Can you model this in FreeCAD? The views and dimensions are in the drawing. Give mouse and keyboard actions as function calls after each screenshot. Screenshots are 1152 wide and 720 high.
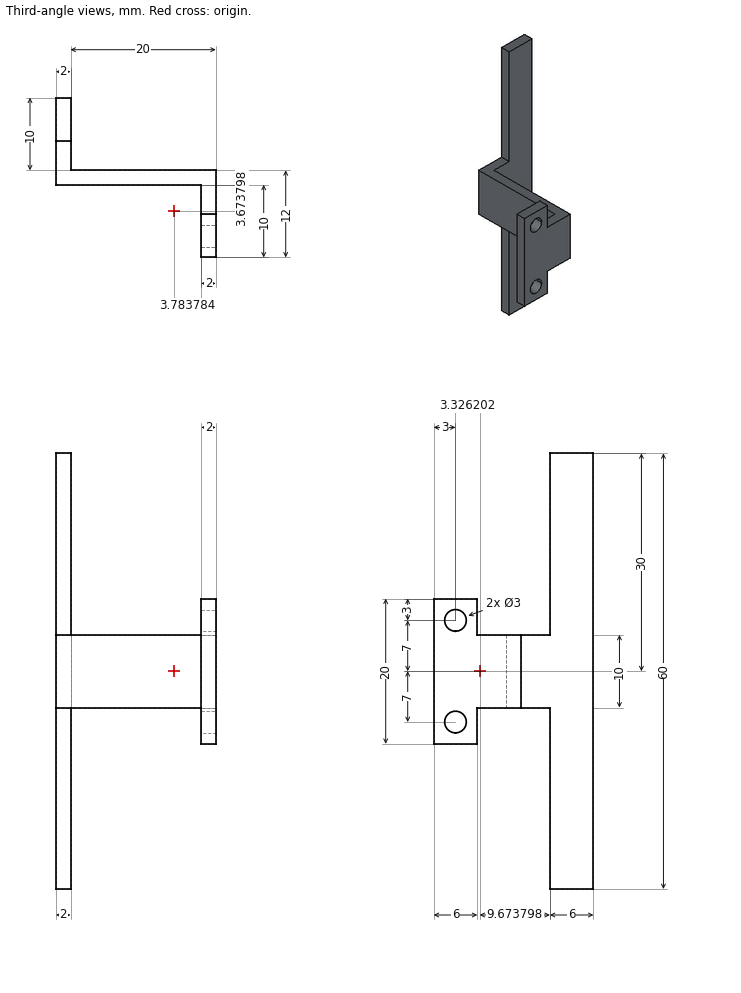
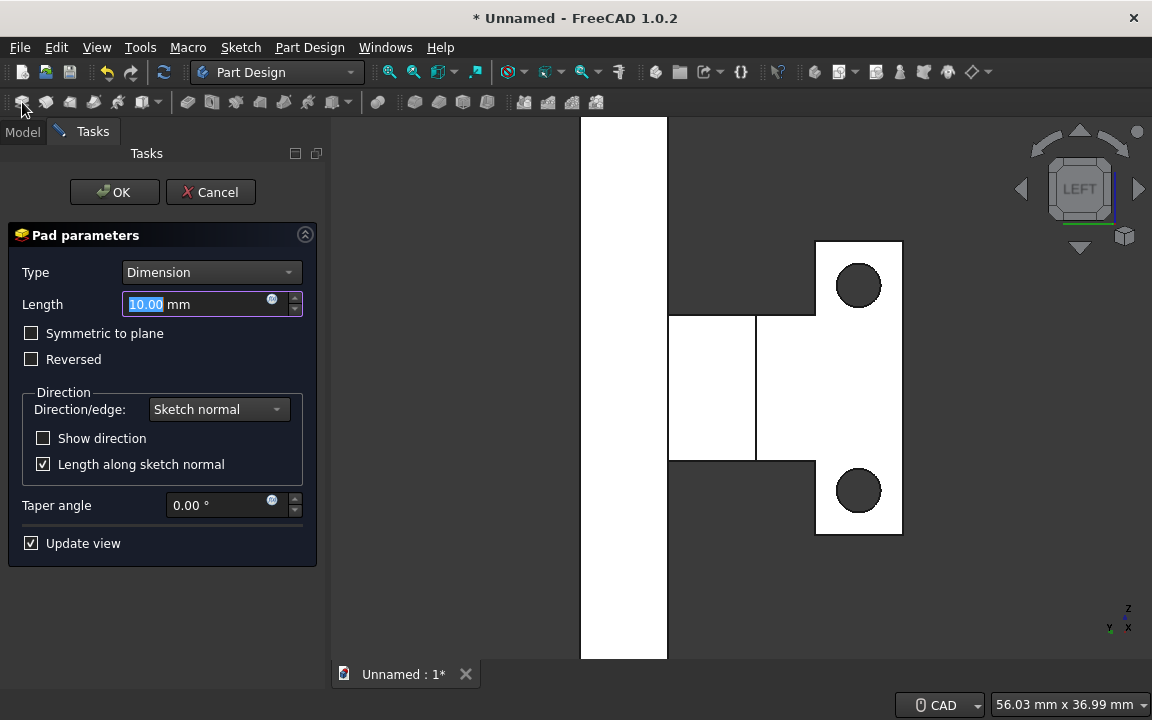
text(2)
key(Tab)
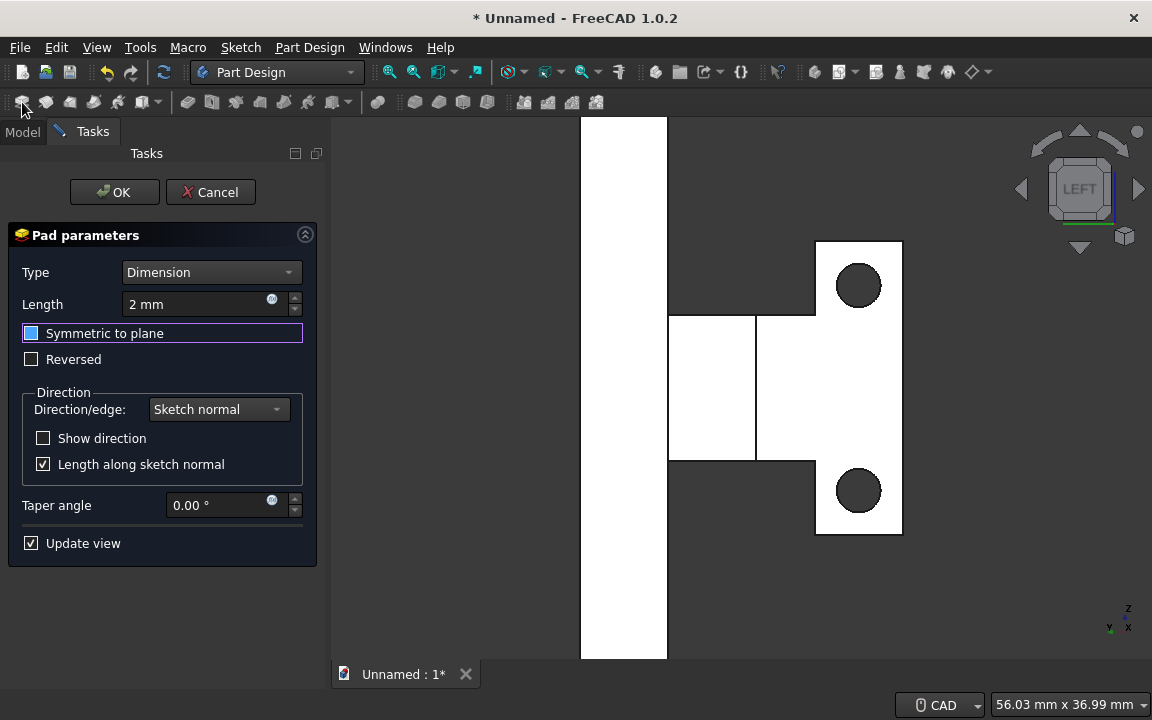
click(30, 359)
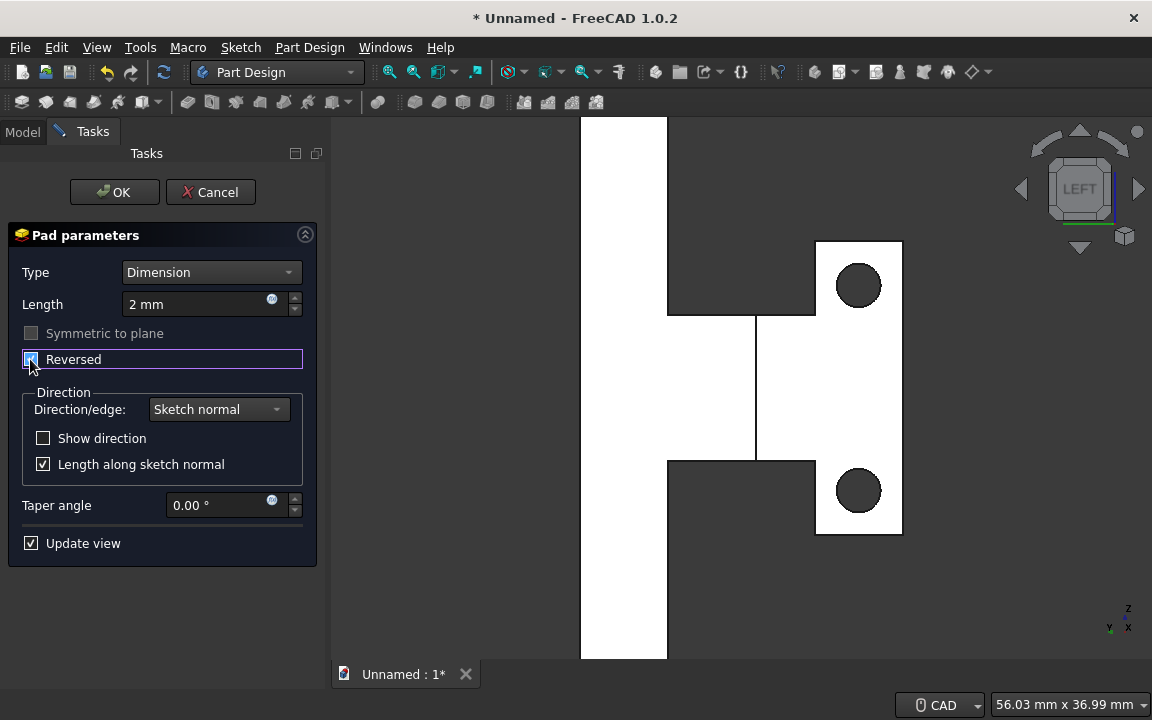
click(115, 192)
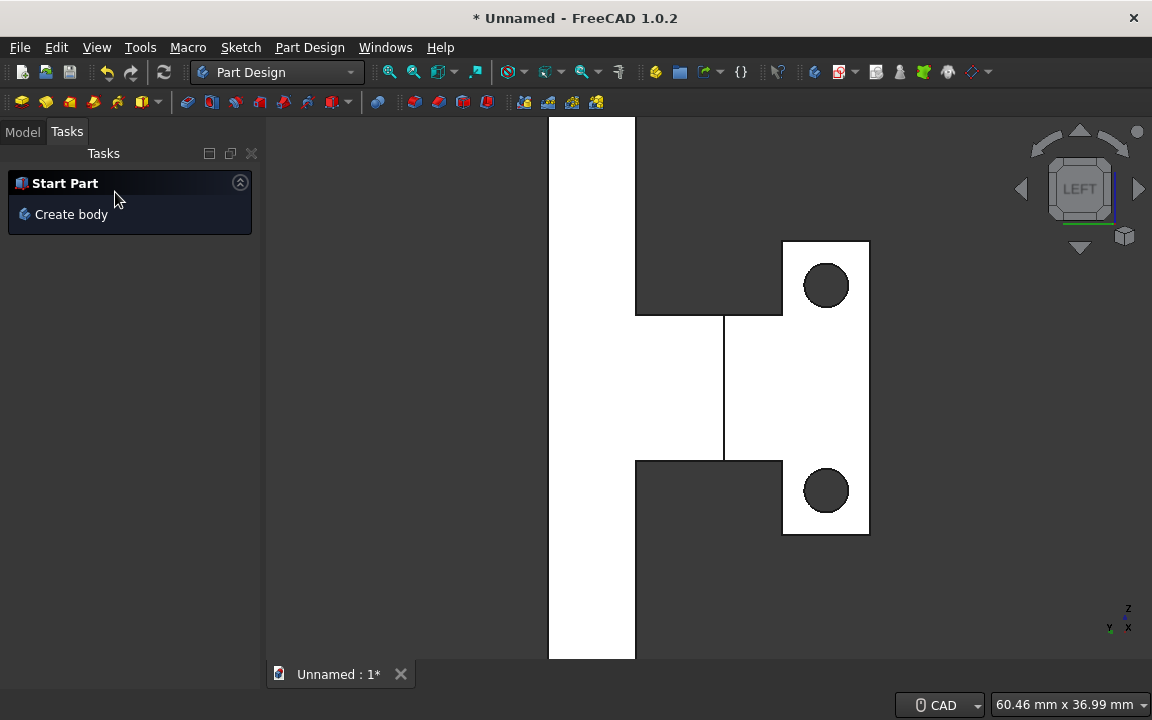
key(0)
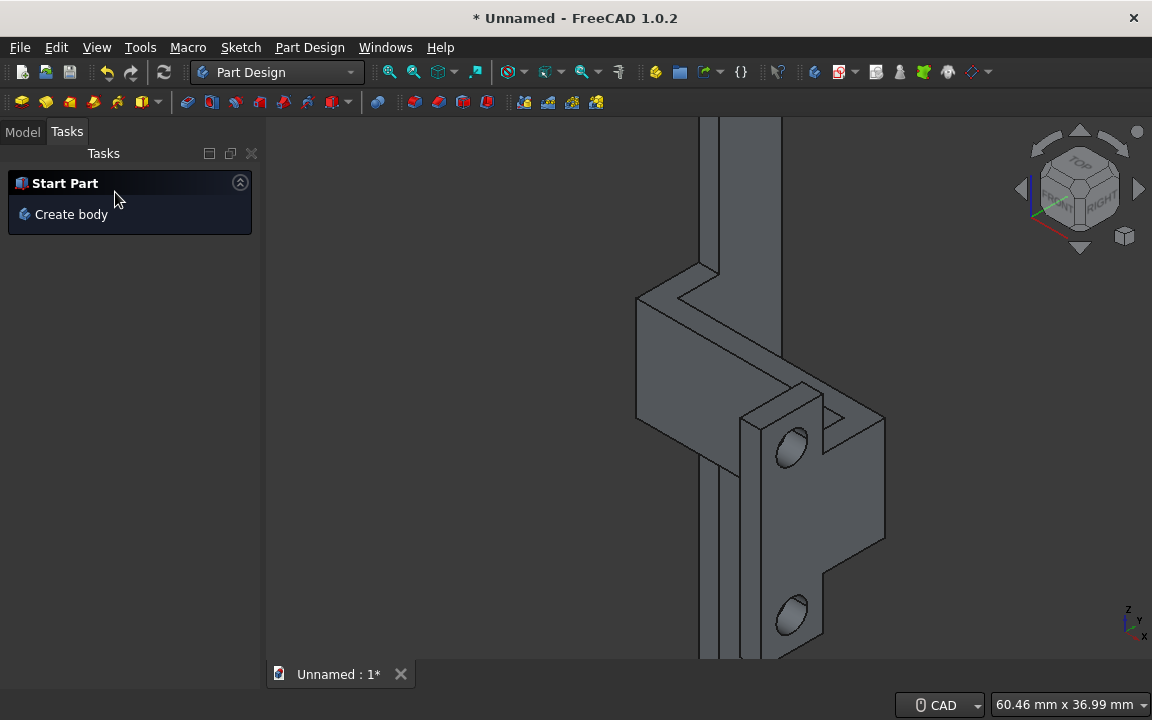
click(390, 72)